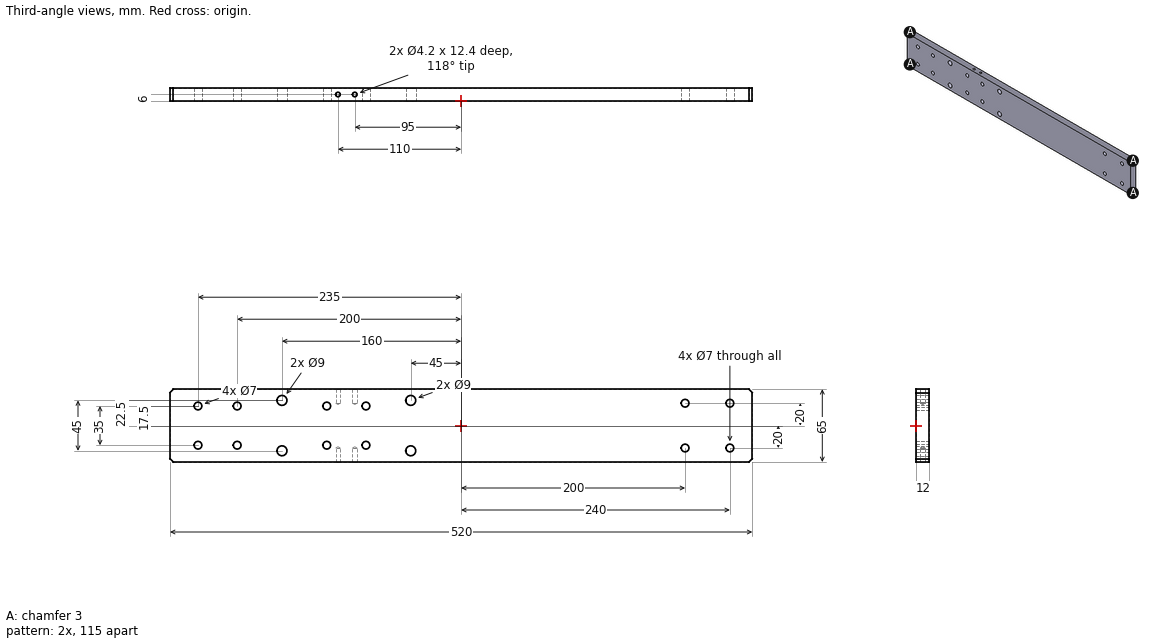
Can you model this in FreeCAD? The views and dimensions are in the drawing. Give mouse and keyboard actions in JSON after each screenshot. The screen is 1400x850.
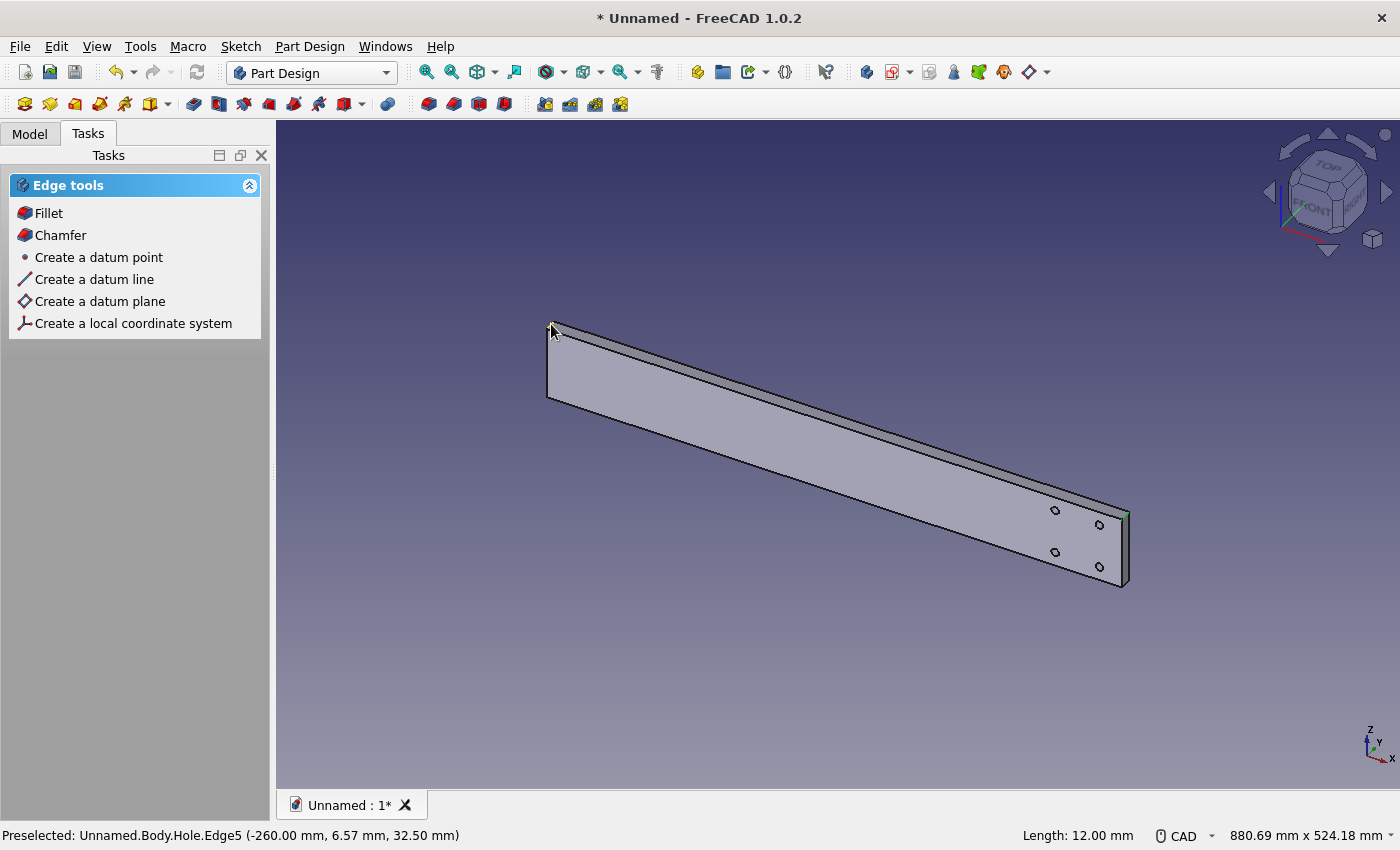
{"action": "key", "text": "0"}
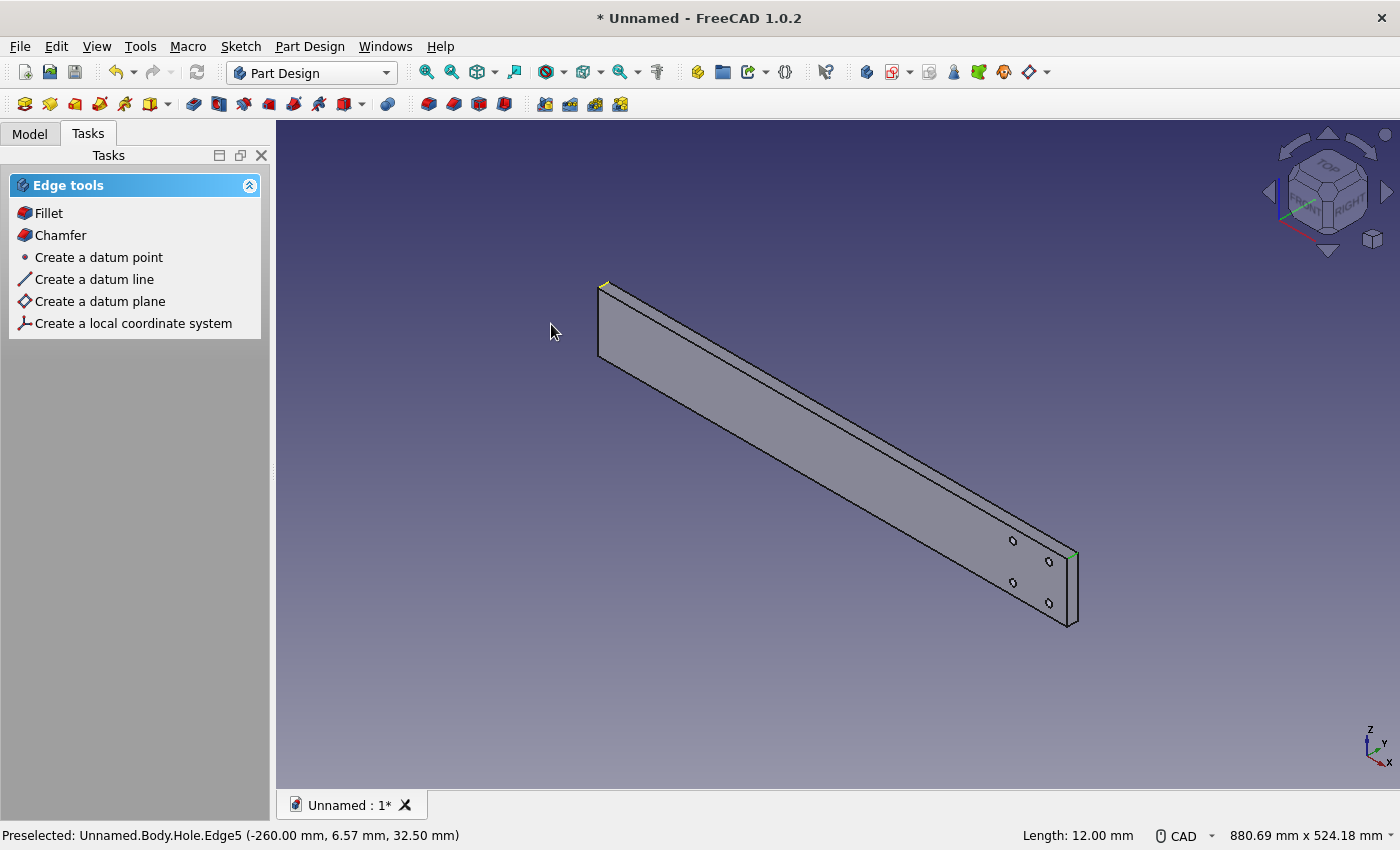
{"action": "scroll", "coordinate": [603, 284], "scroll_direction": "up", "scroll_amount": 5}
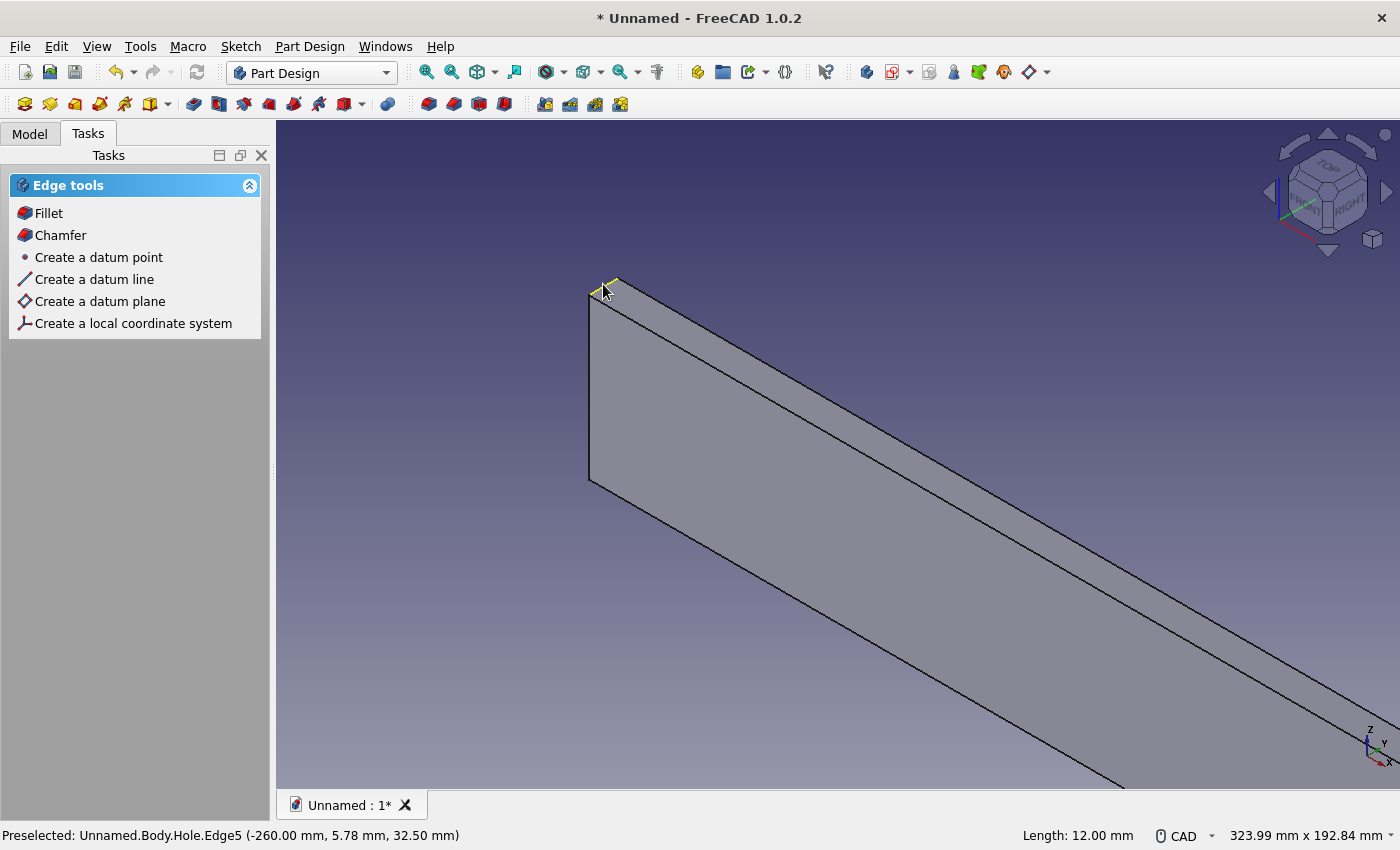
{"action": "key", "text": "v f"}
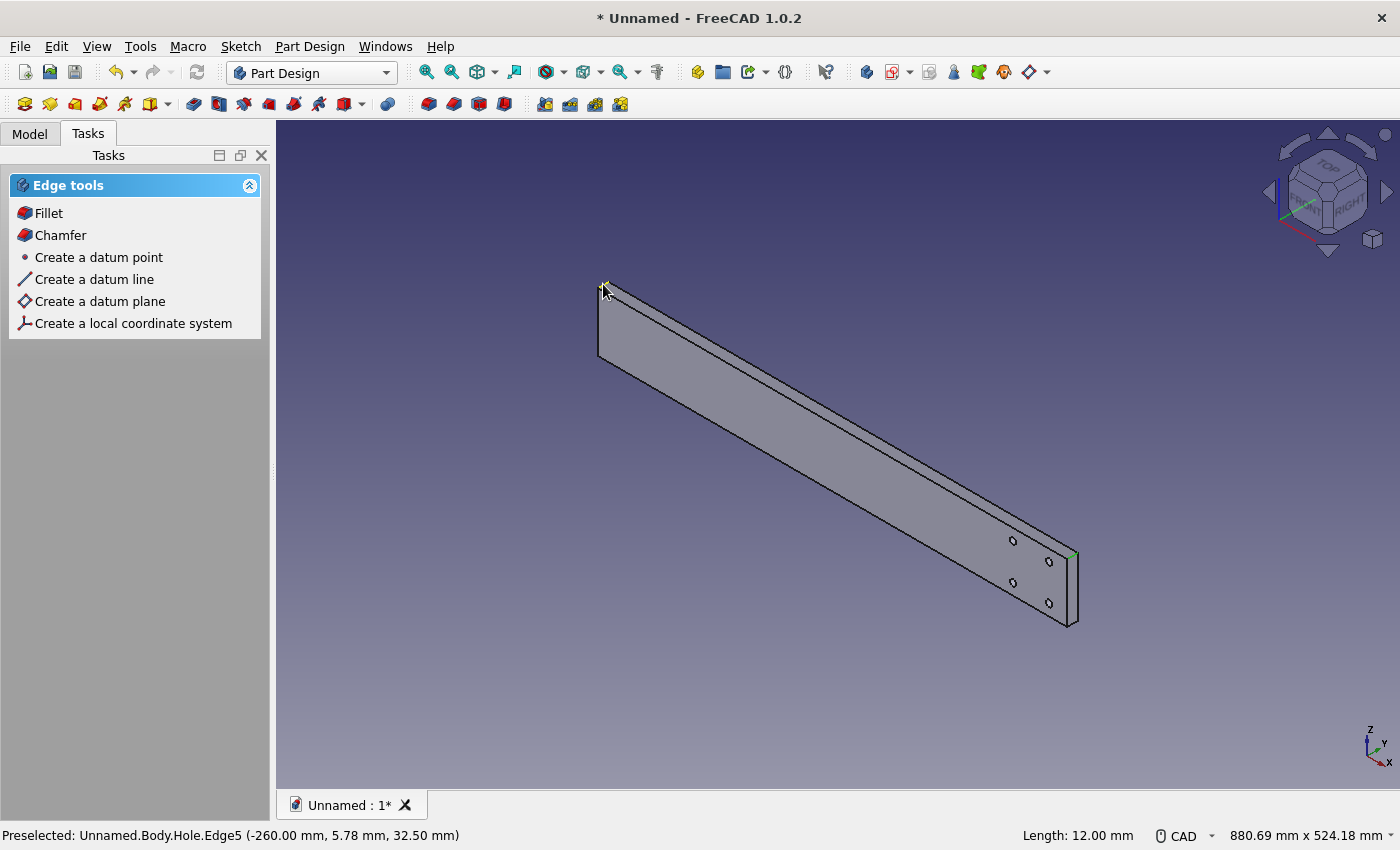
{"action": "key", "text": "2"}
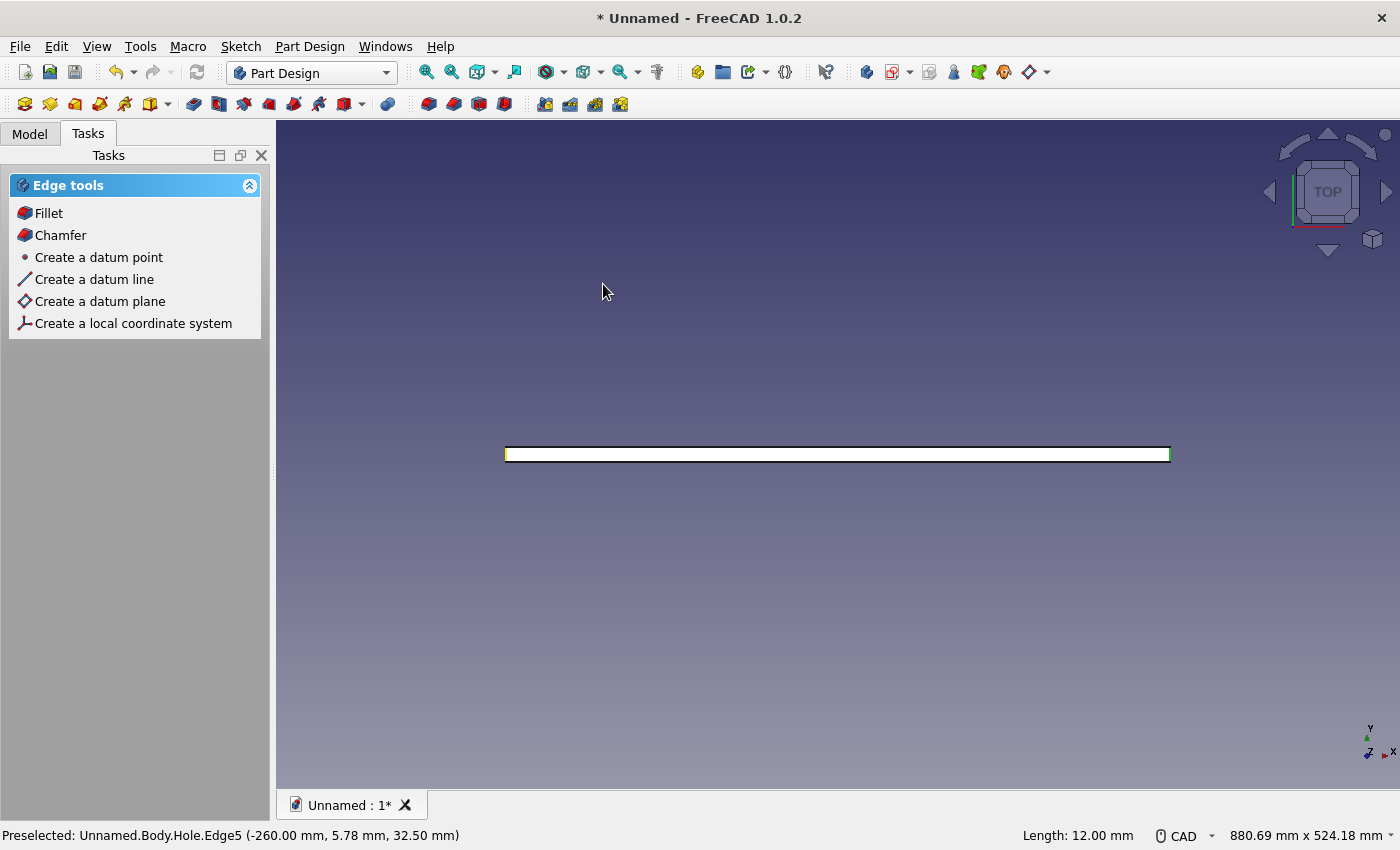
{"action": "left_click", "coordinate": [506, 453], "text": "ctrl"}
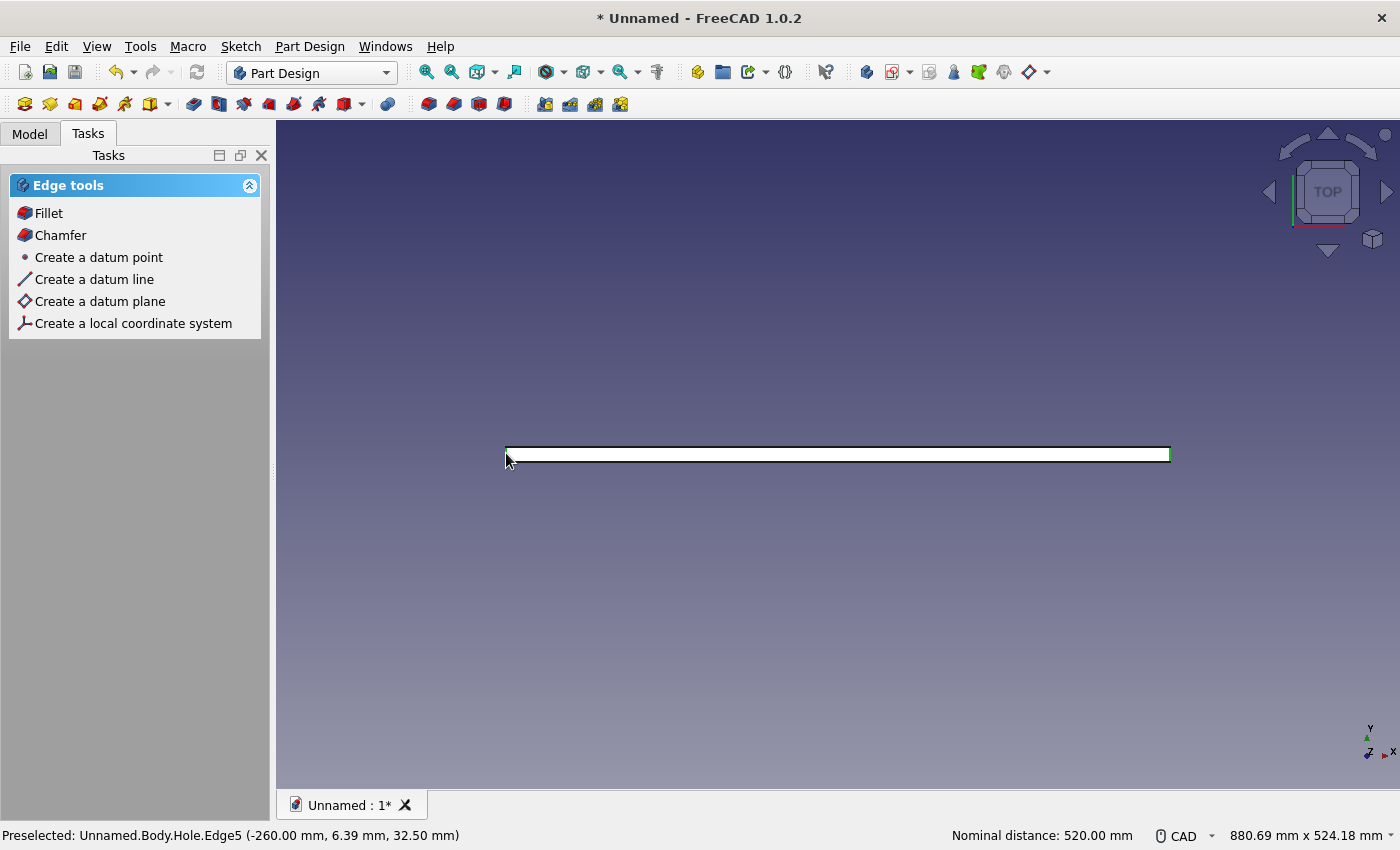
{"action": "scroll", "coordinate": [506, 453], "scroll_direction": "up", "scroll_amount": 5}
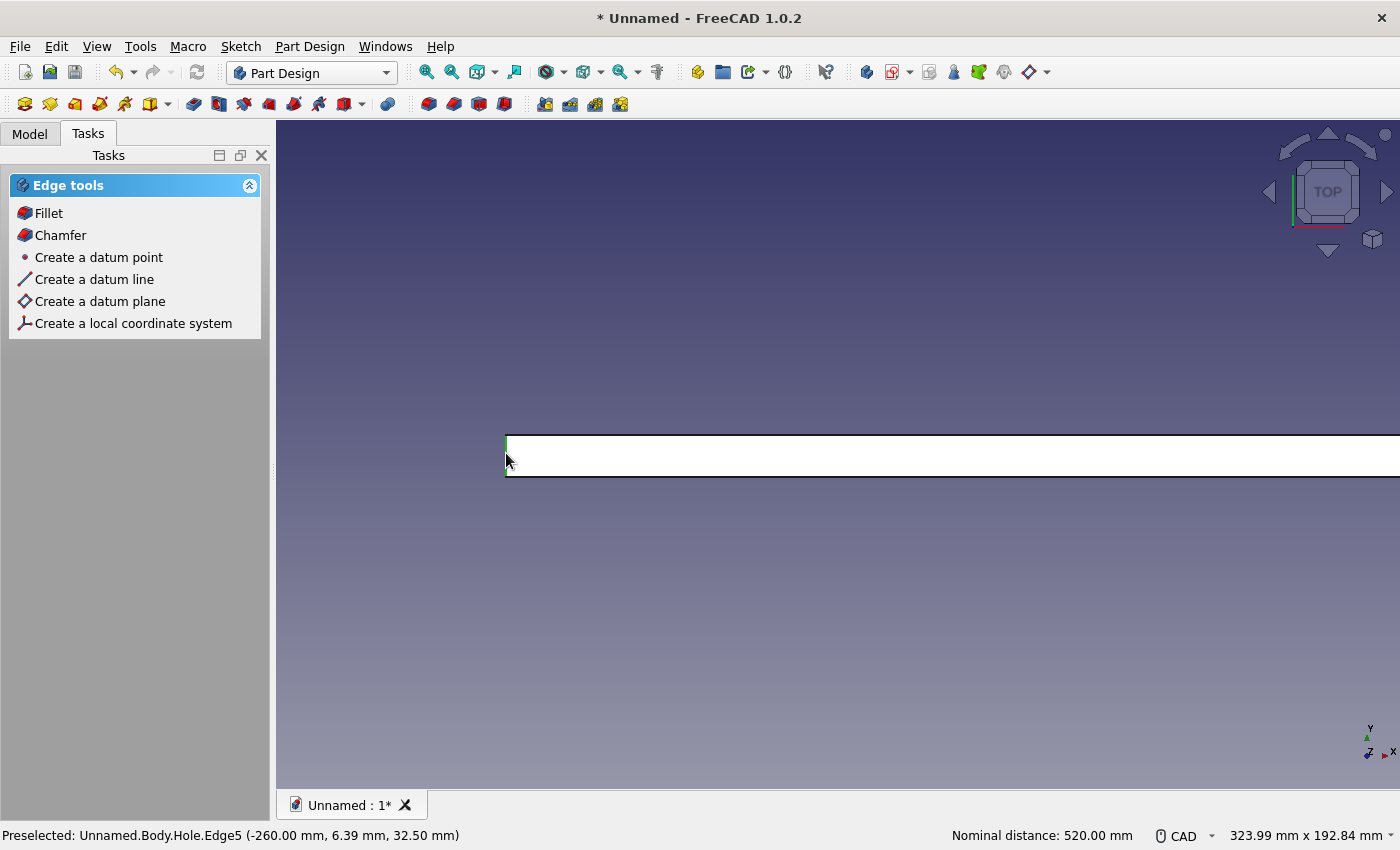
{"action": "left_click", "coordinate": [427, 72]}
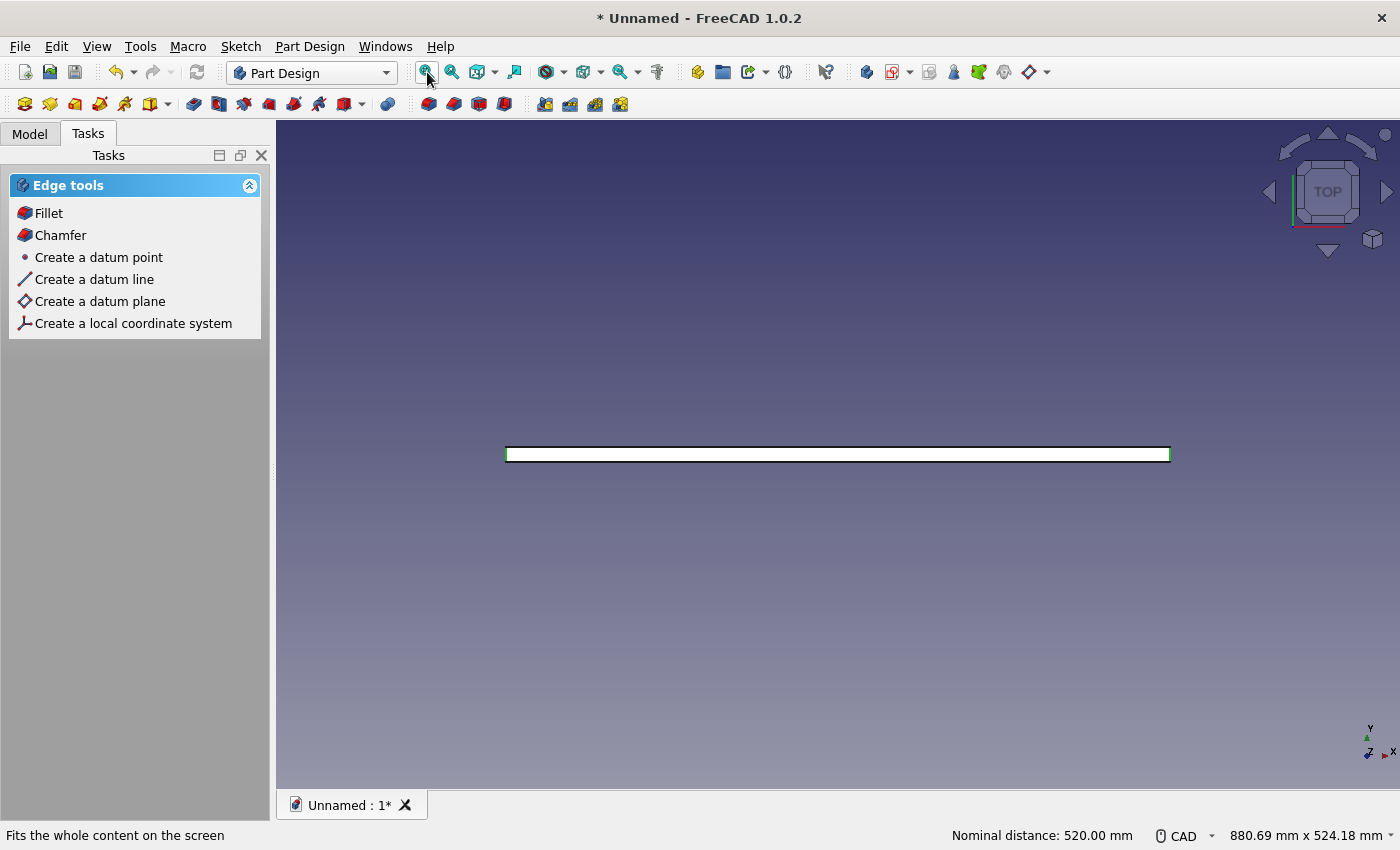
{"action": "key", "text": "1"}